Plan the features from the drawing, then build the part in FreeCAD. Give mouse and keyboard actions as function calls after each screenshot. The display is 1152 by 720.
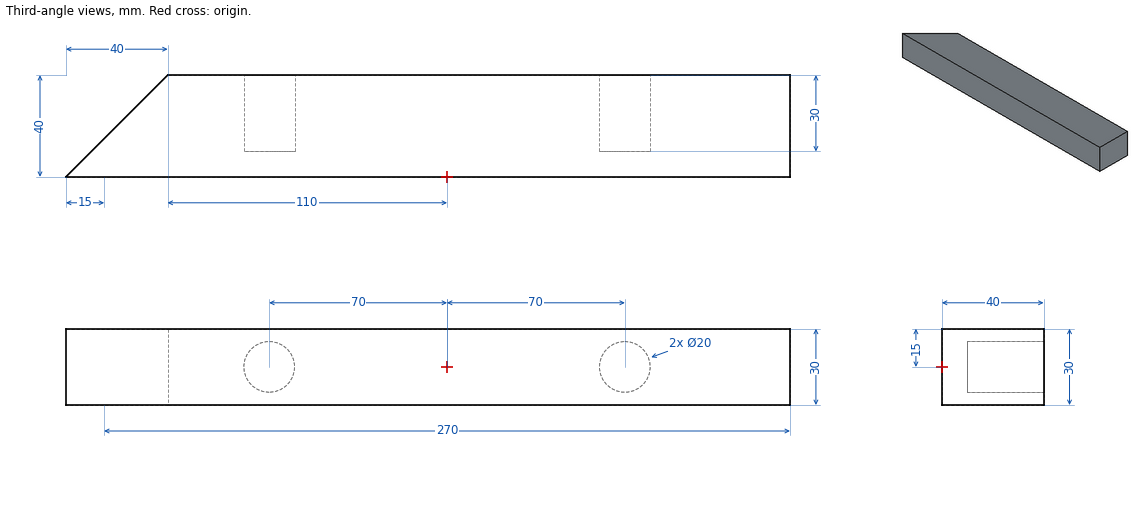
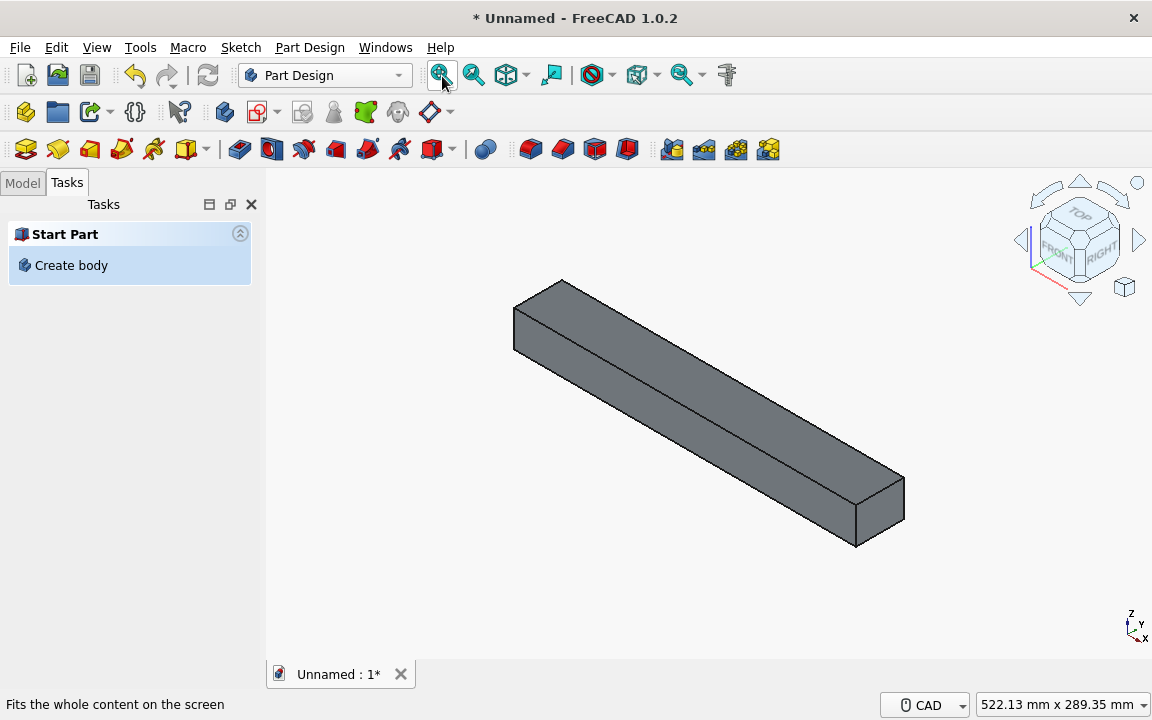
click(856, 476)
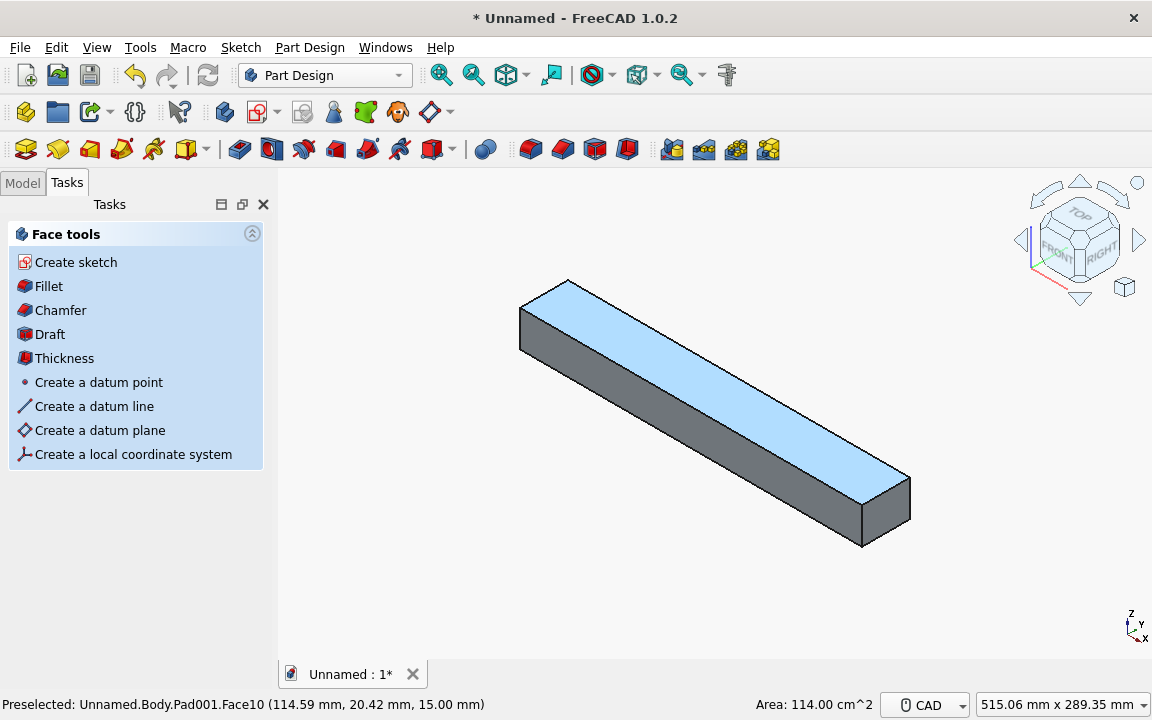
click(258, 112)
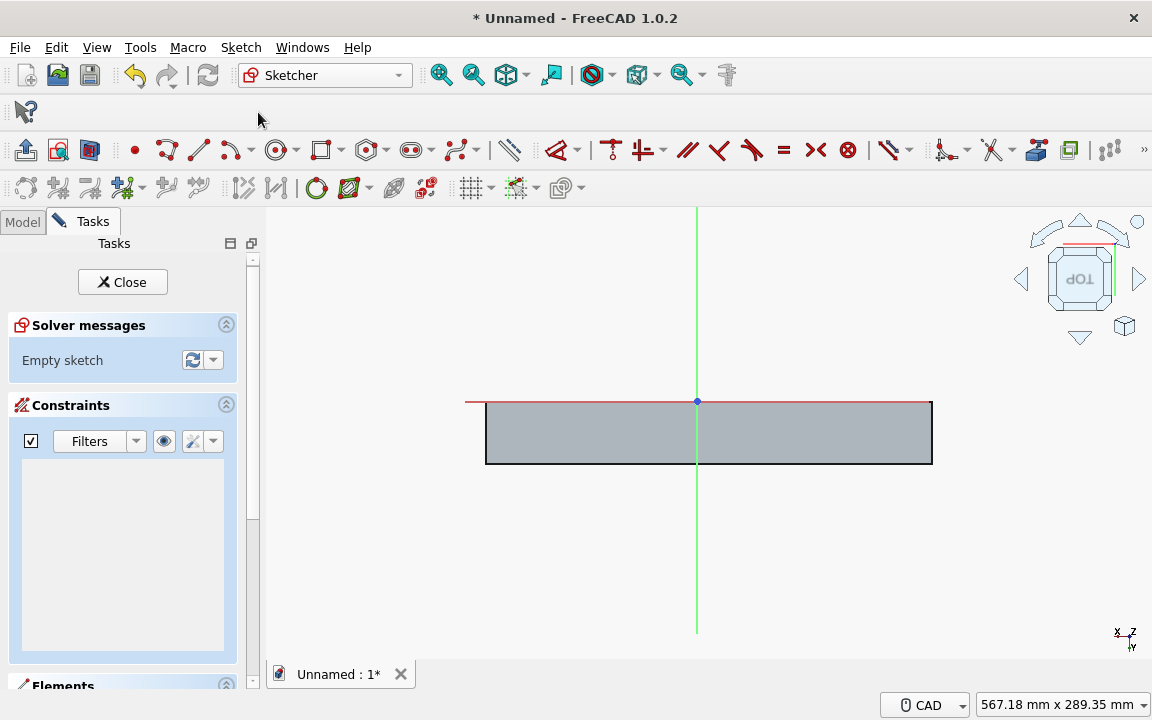
scroll(985, 433, up, 7)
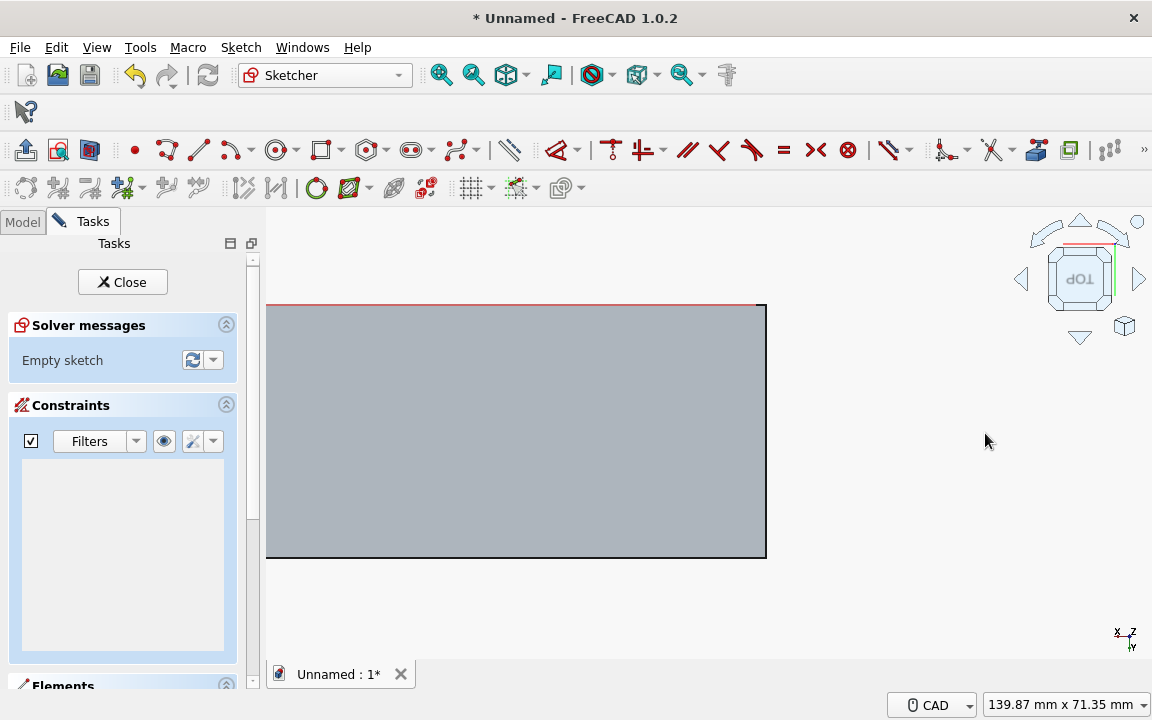
click(168, 150)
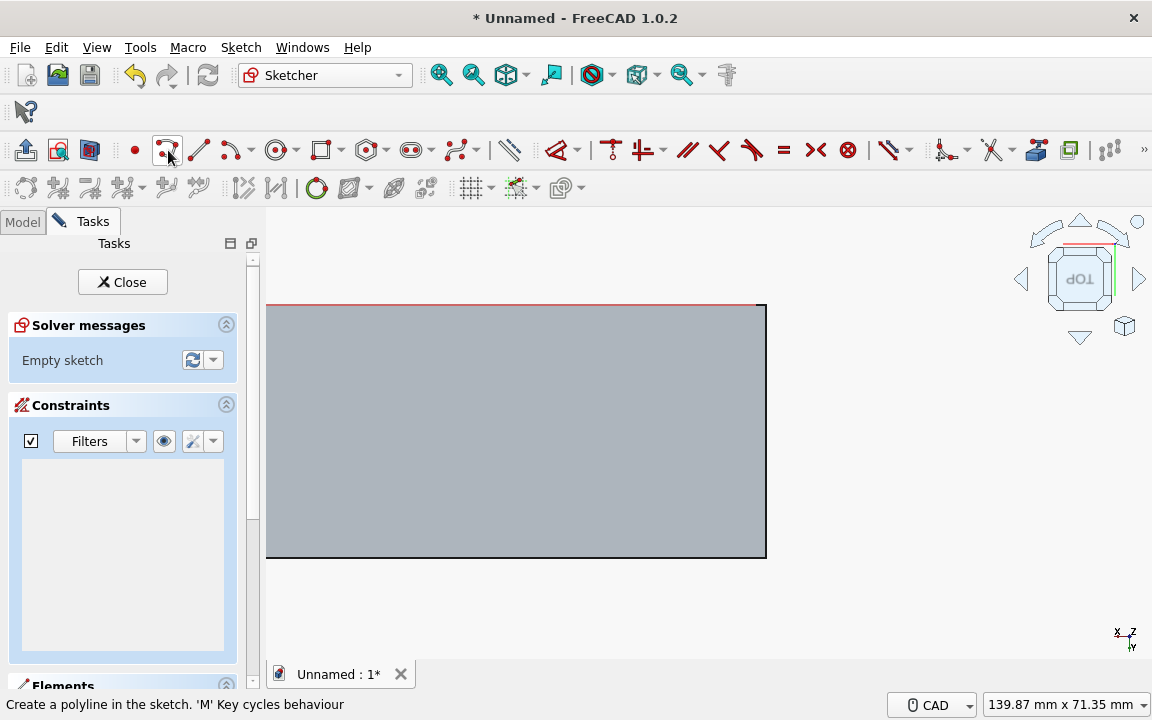
click(513, 558)
click(766, 558)
click(766, 305)
click(513, 559)
key(Escape)
key(Escape)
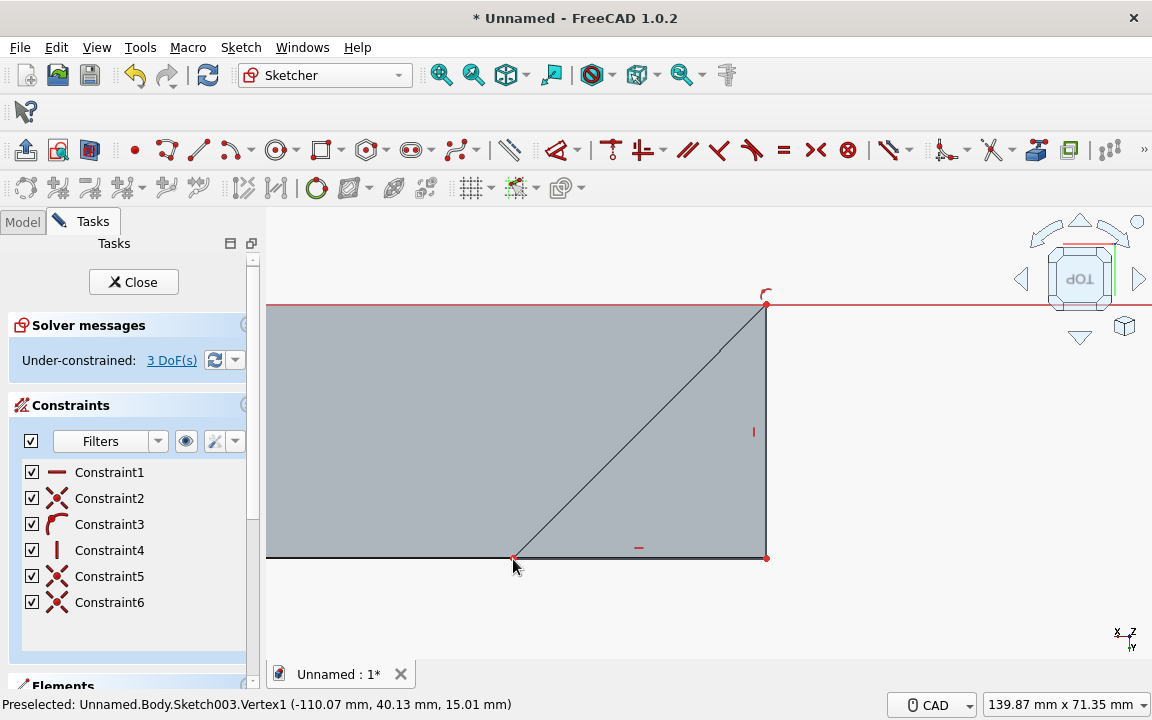
key(d)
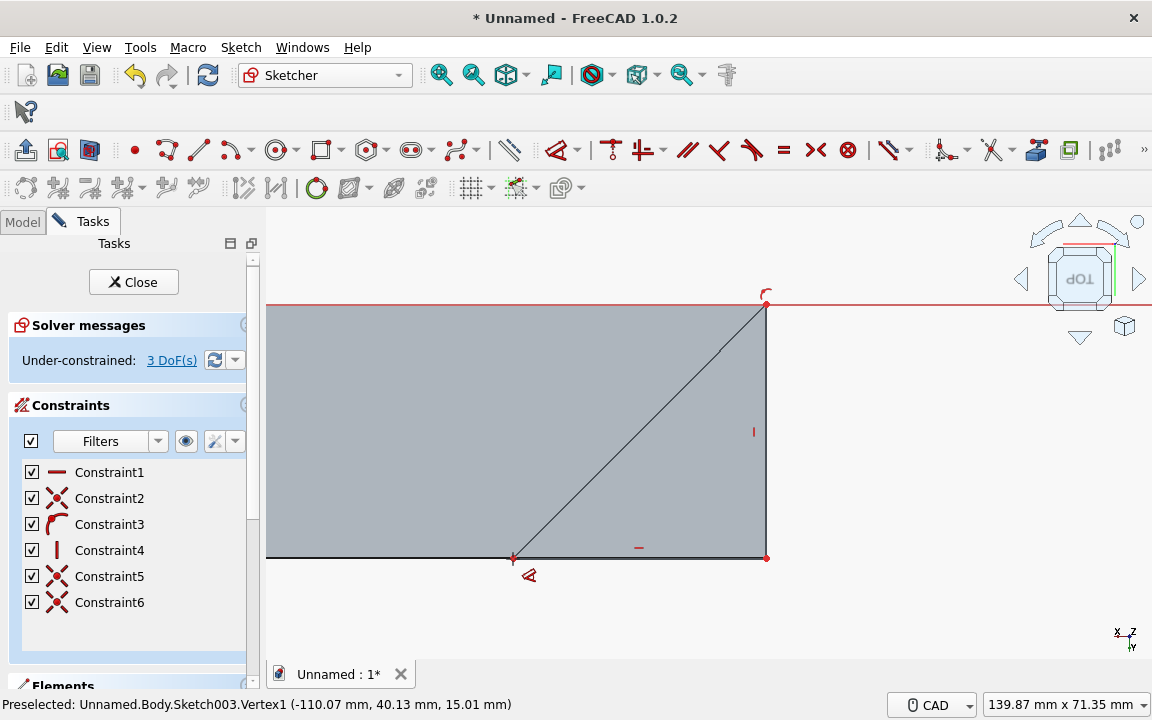
click(589, 559)
click(640, 593)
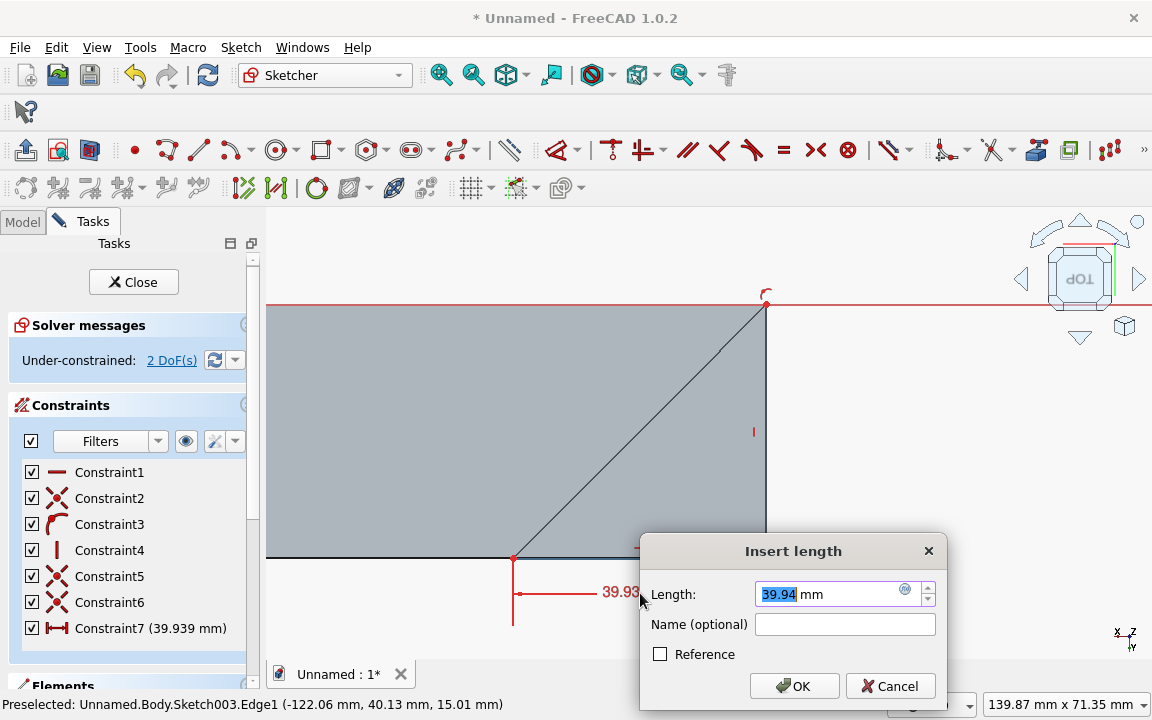
text(40)
key(Return)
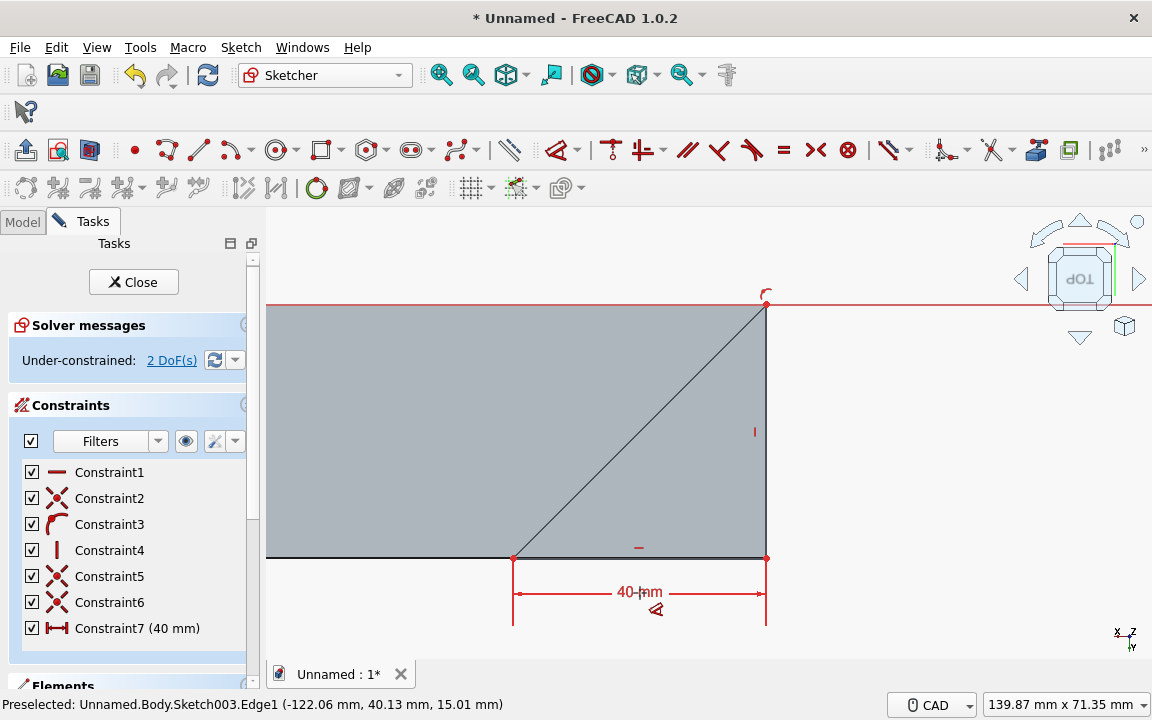
click(766, 483)
click(800, 432)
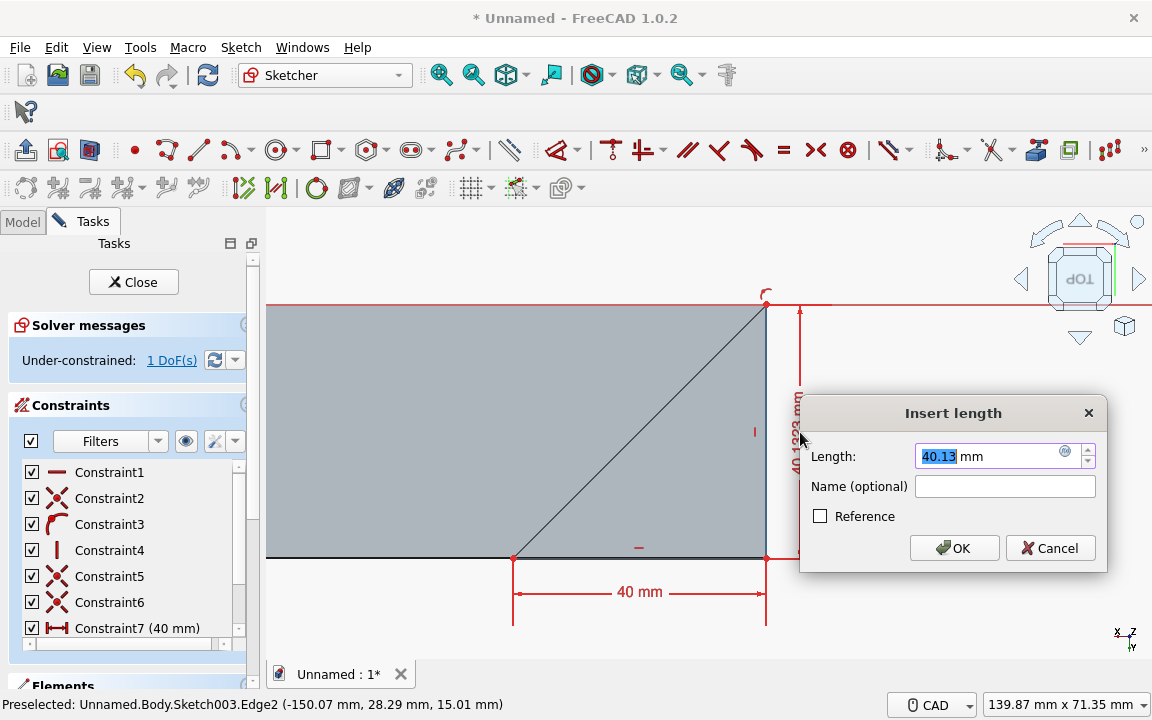
text(40)
key(Return)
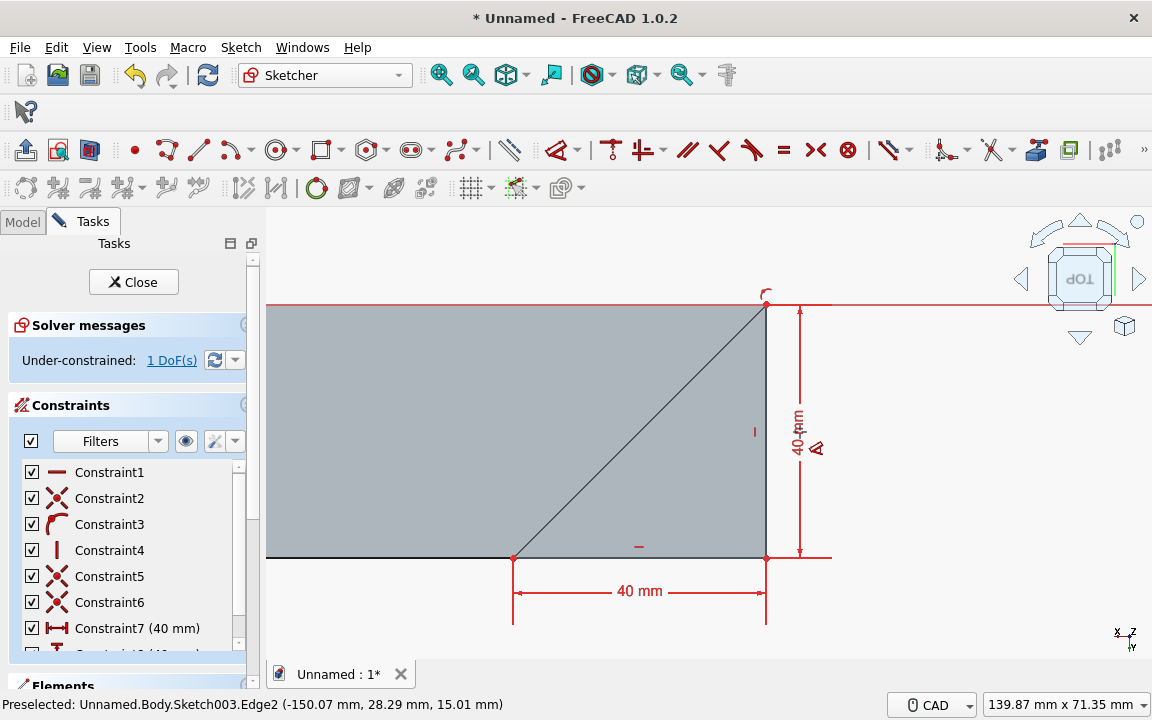
click(513, 558)
click(404, 271)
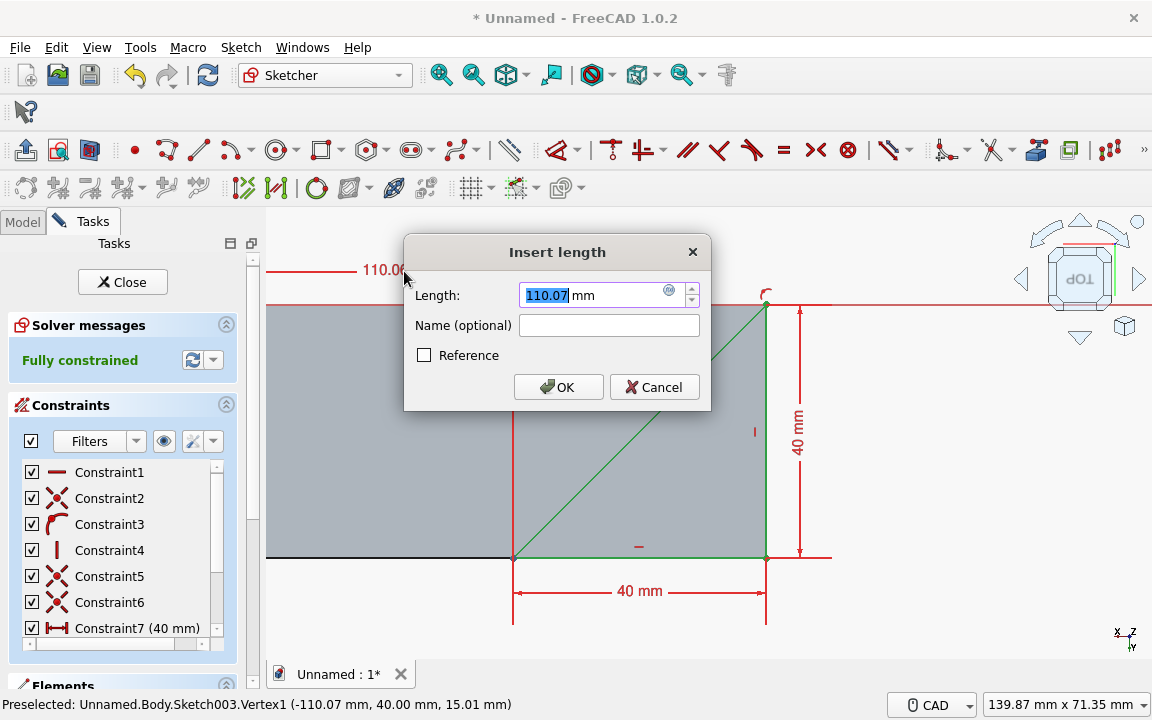
text(110)
key(Return)
key(Escape)